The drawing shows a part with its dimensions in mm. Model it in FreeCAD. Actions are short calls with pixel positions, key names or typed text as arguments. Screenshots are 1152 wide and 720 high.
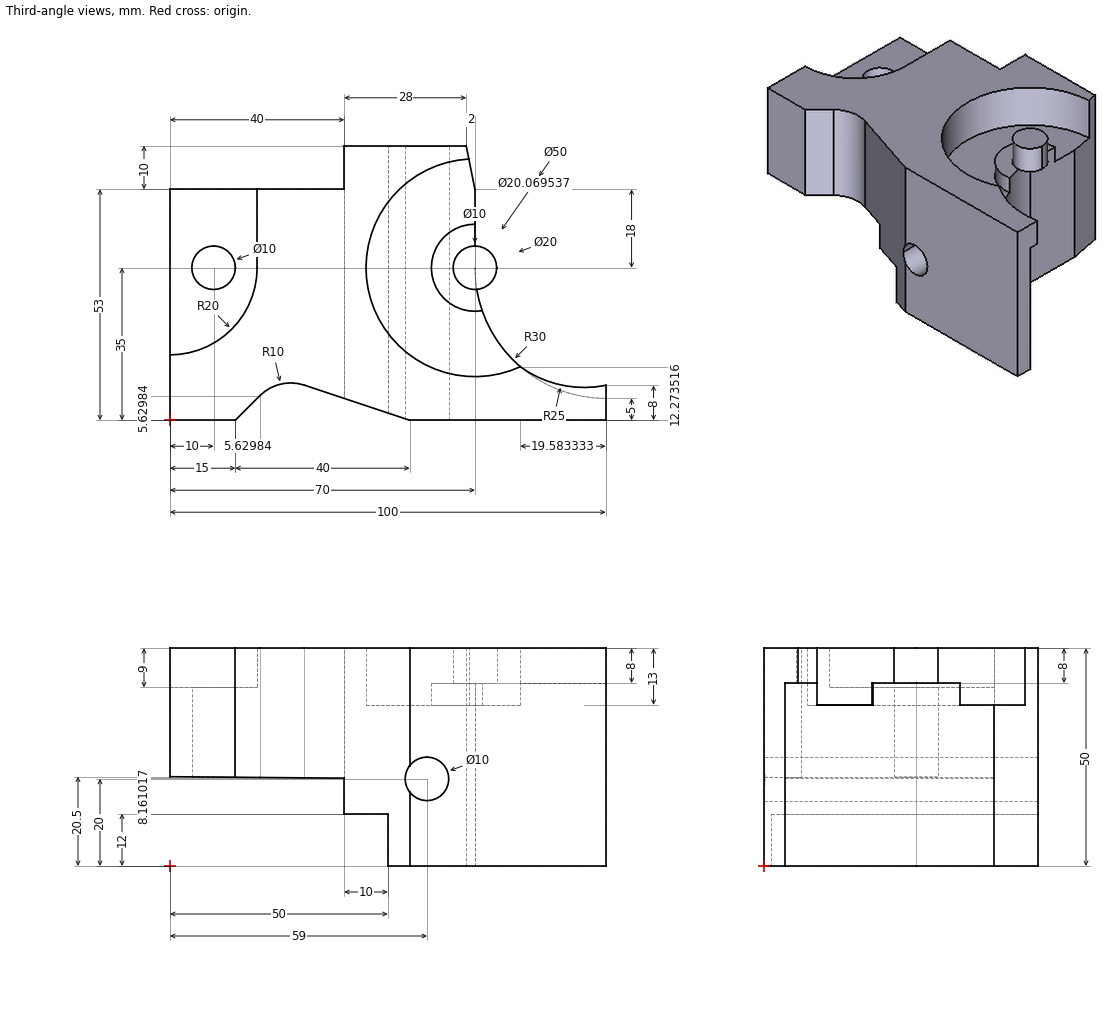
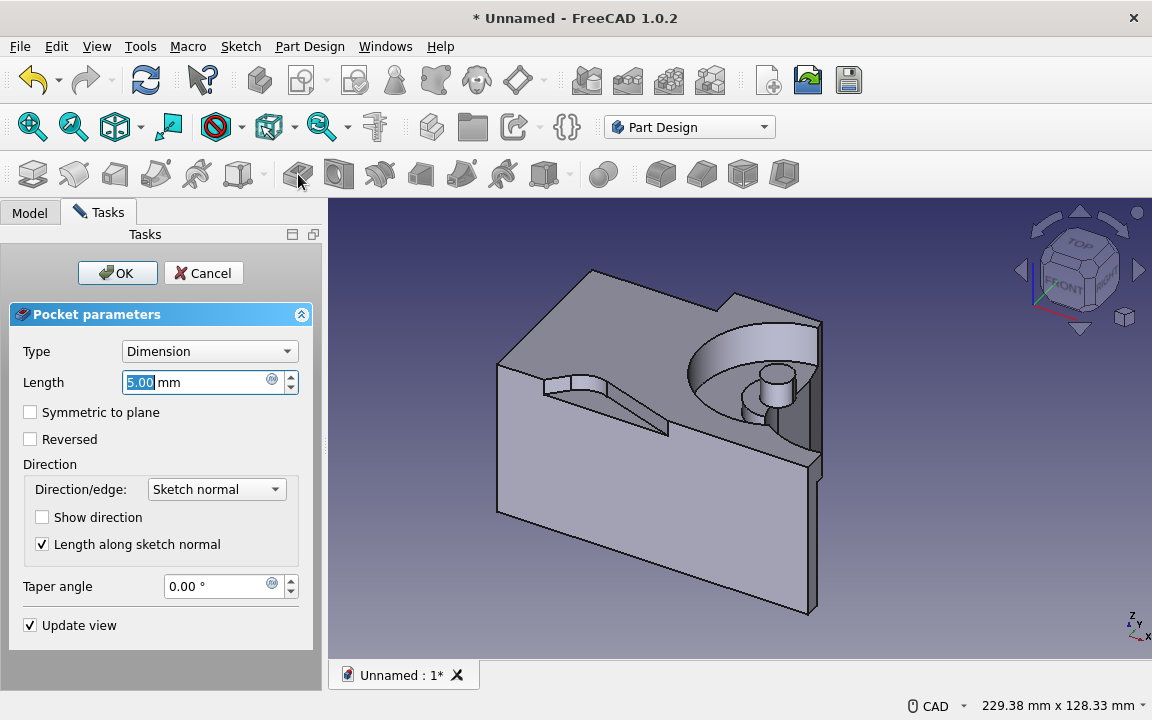
click(210, 352)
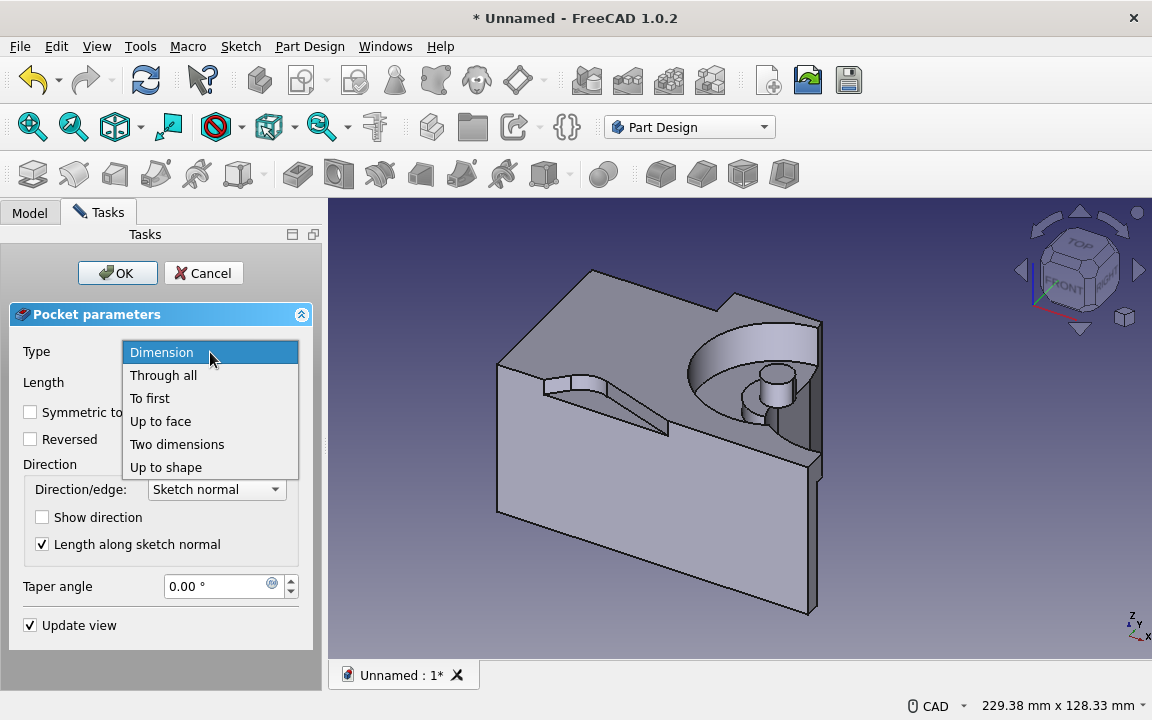
click(208, 376)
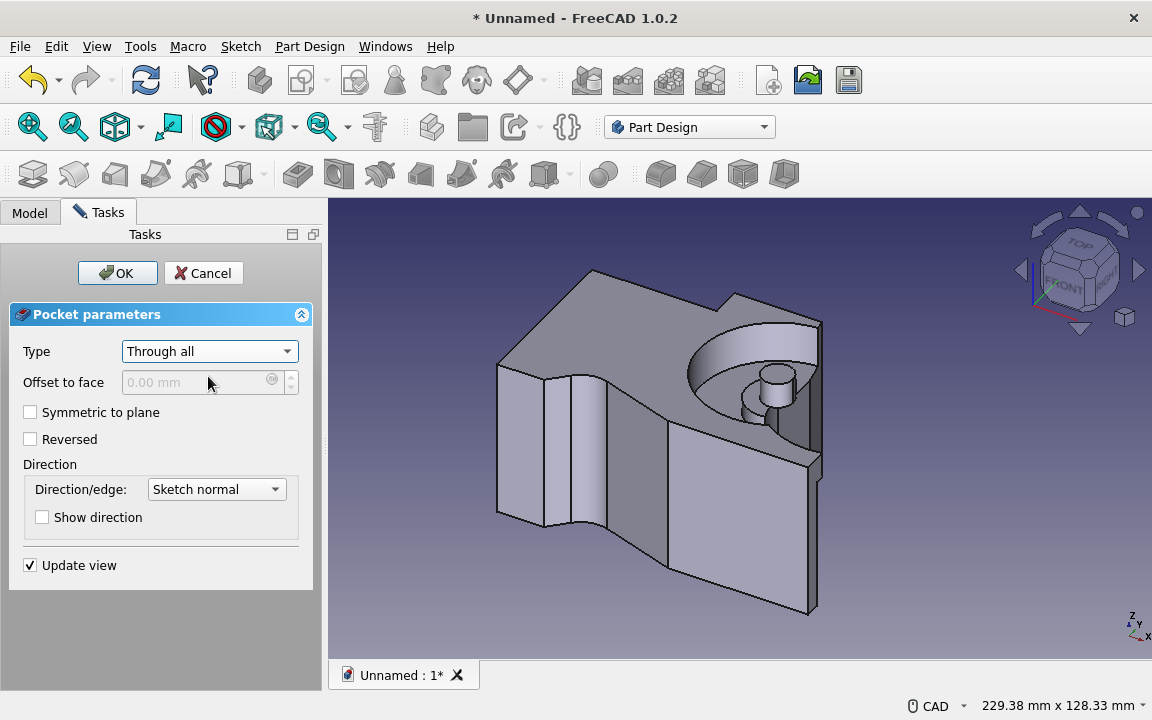
click(118, 273)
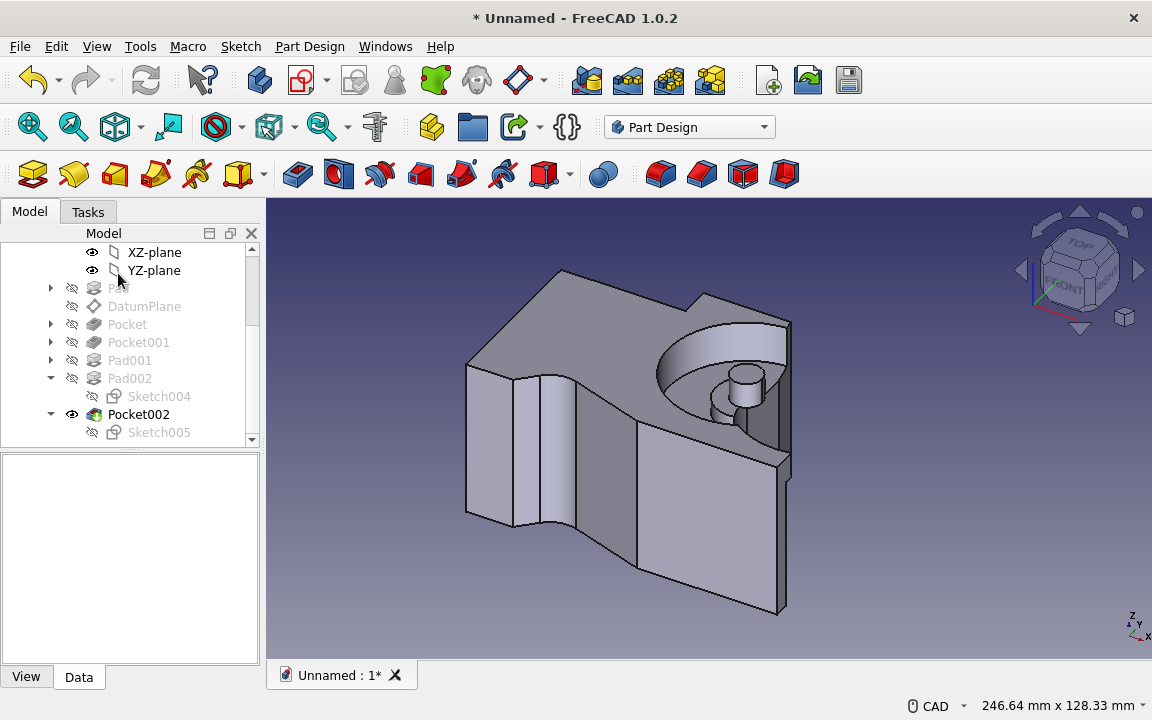
click(589, 329)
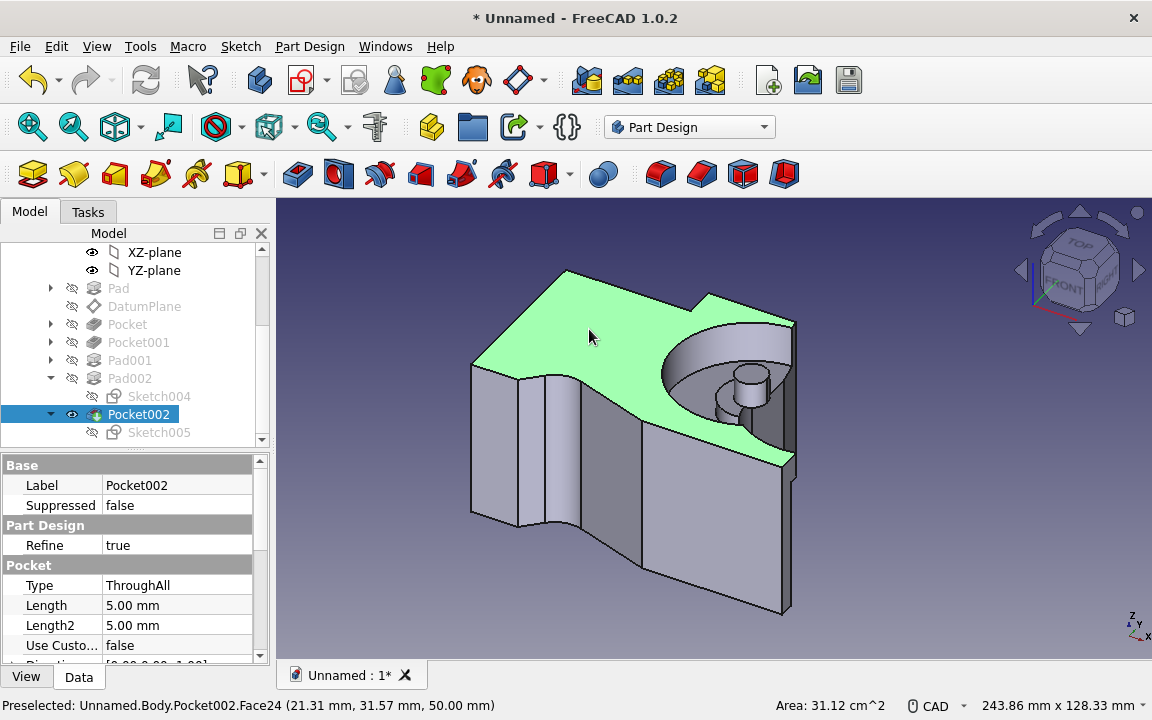
click(300, 80)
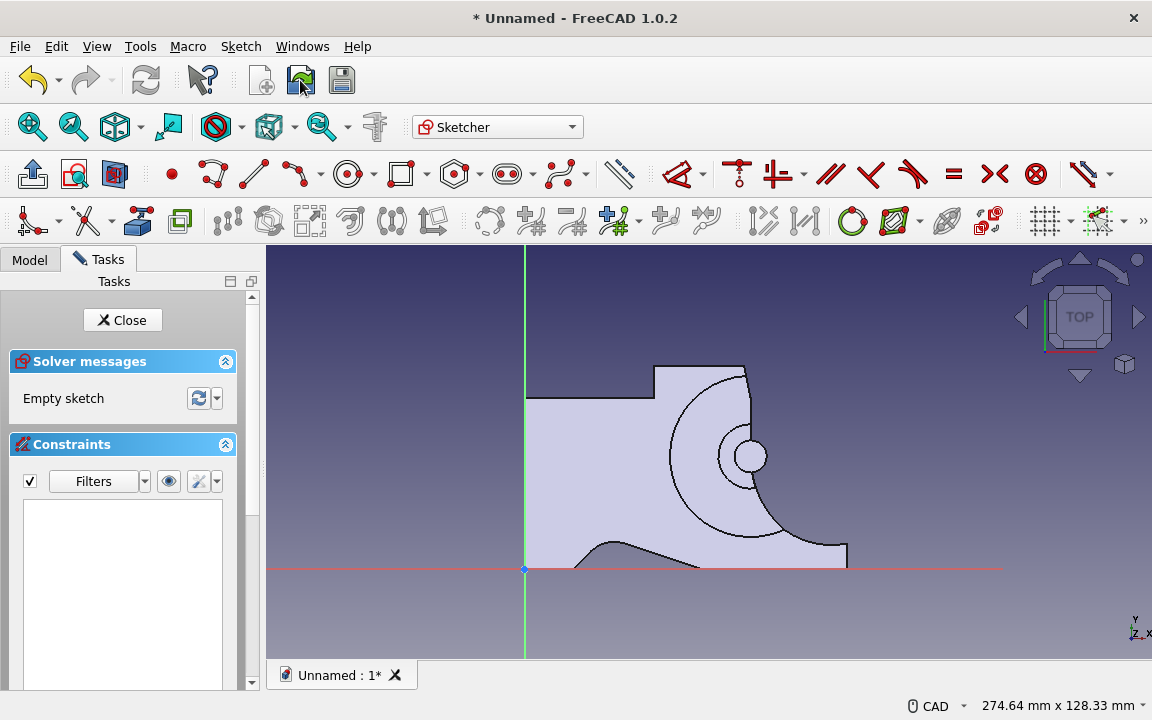
scroll(387, 549, up, 2)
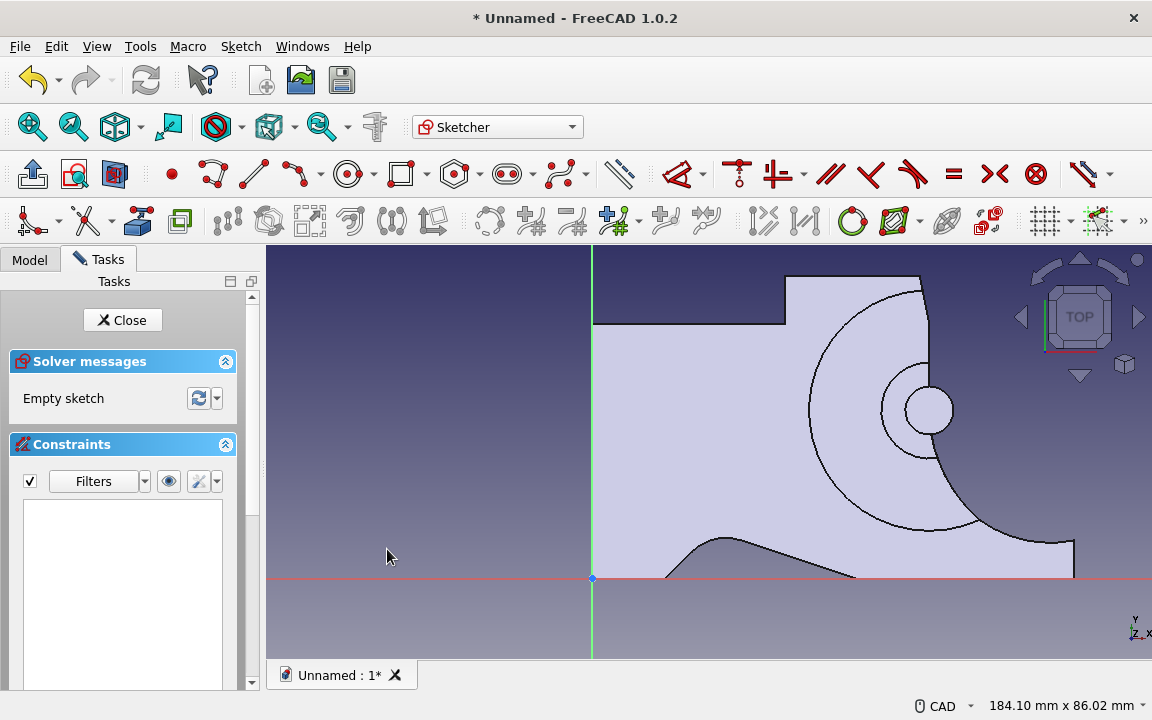
key(g)
key(m)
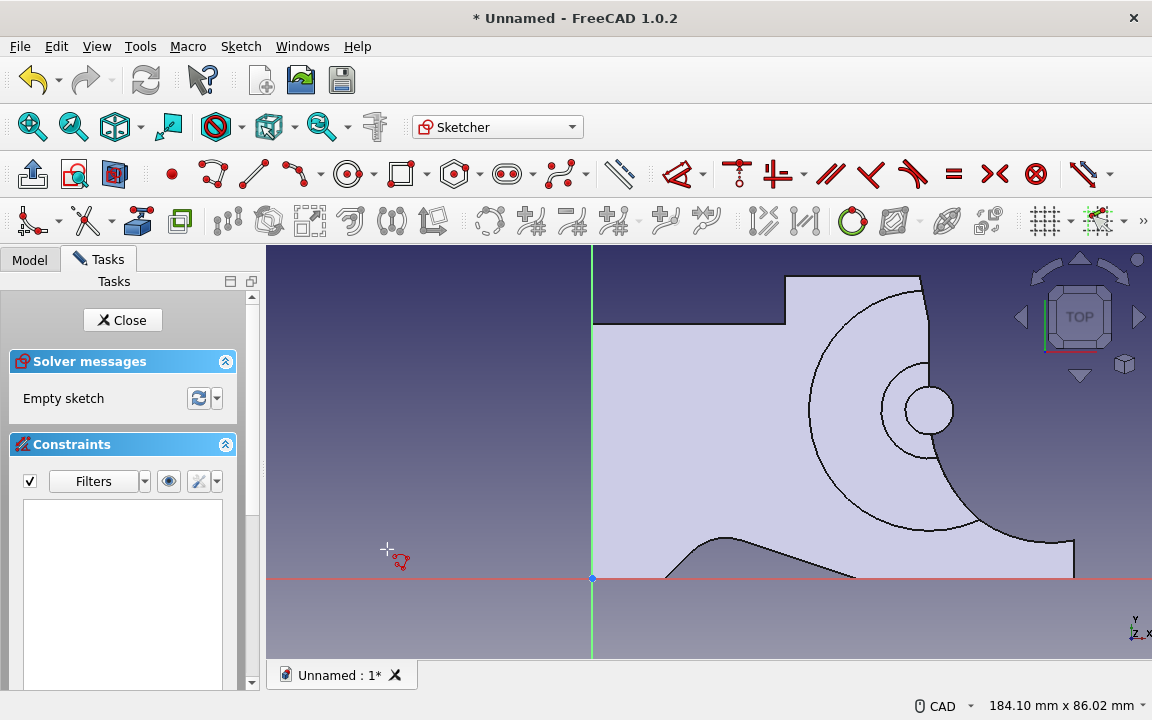
click(689, 411)
click(689, 324)
click(592, 324)
click(601, 507)
right_click(601, 507)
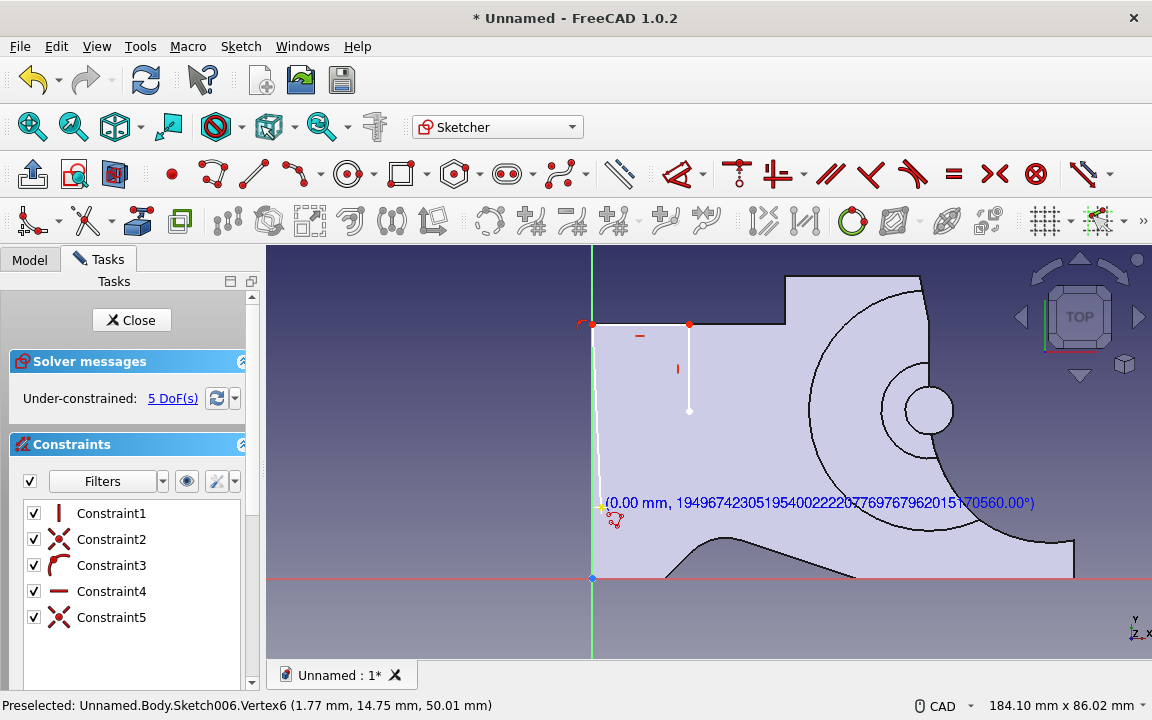
key(g)
key(3)
key(a)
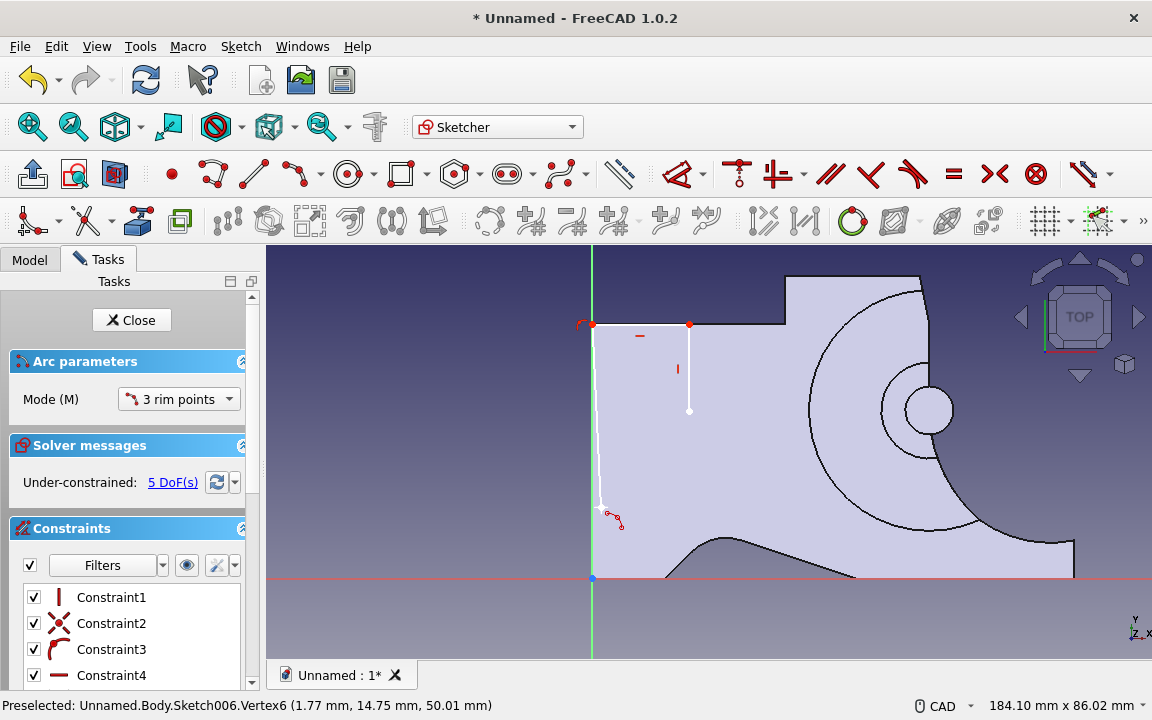
click(601, 508)
click(689, 412)
click(661, 479)
key(Escape)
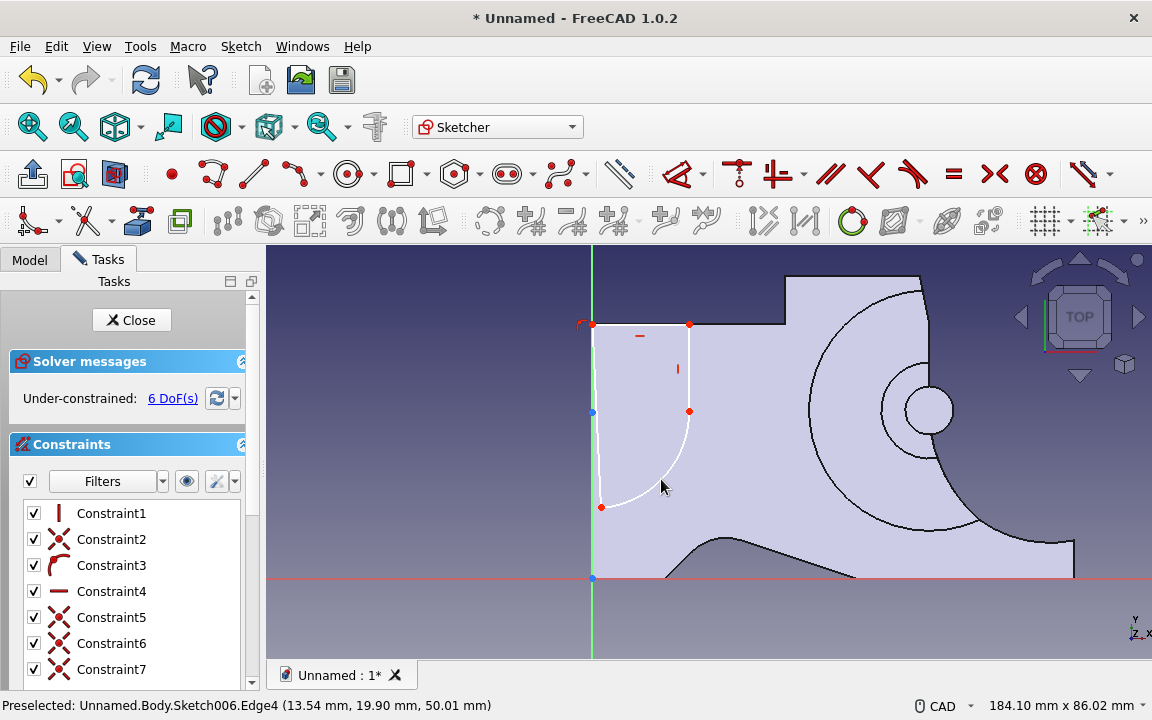
click(689, 386)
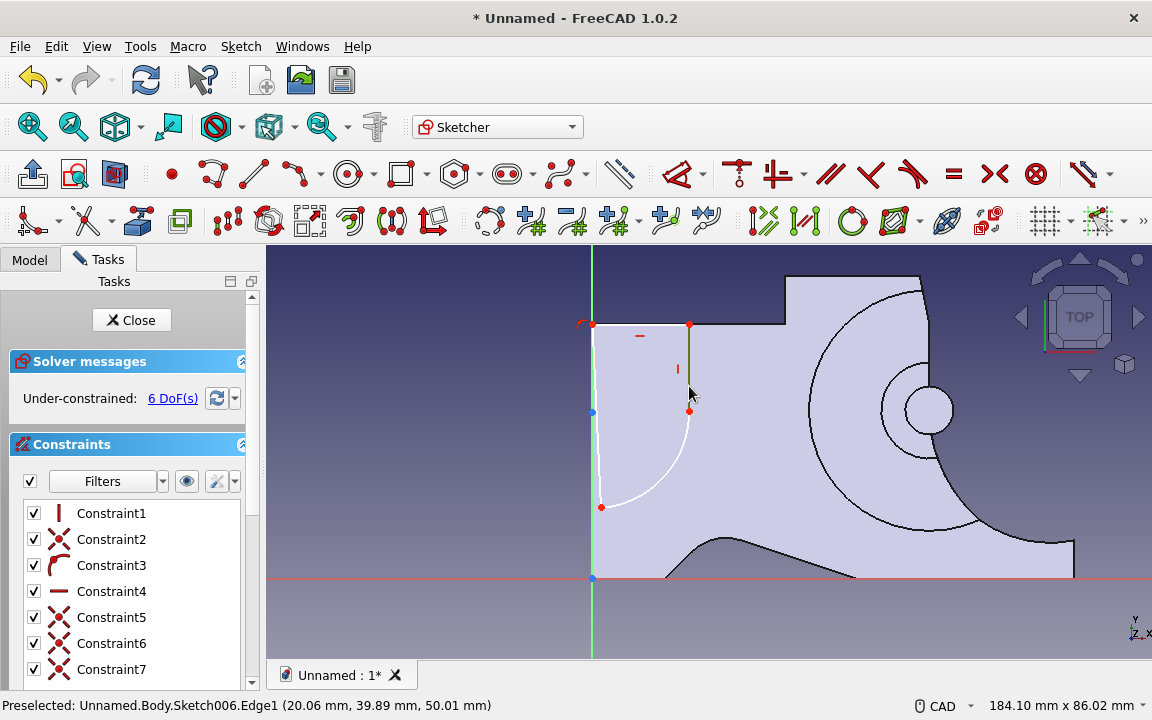
click(642, 495)